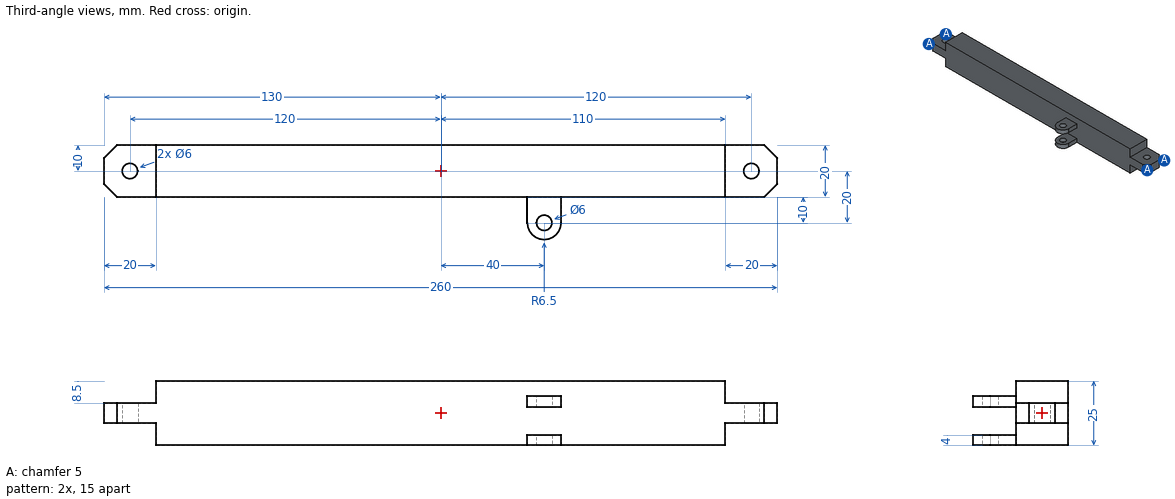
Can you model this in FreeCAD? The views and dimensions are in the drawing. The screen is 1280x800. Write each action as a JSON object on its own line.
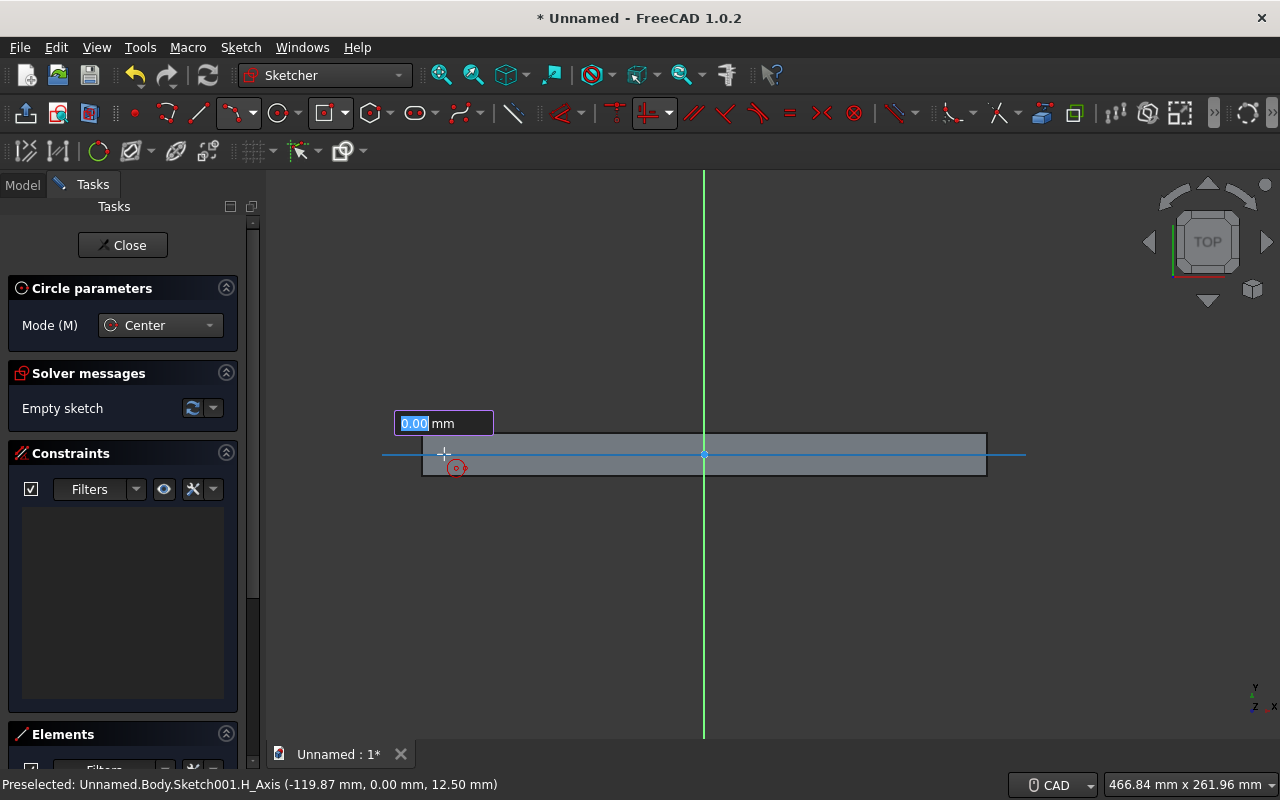
{"action": "scroll", "coordinate": [441, 461], "scroll_direction": "up", "scroll_amount": 5}
{"action": "mouse_move", "coordinate": [442, 459]}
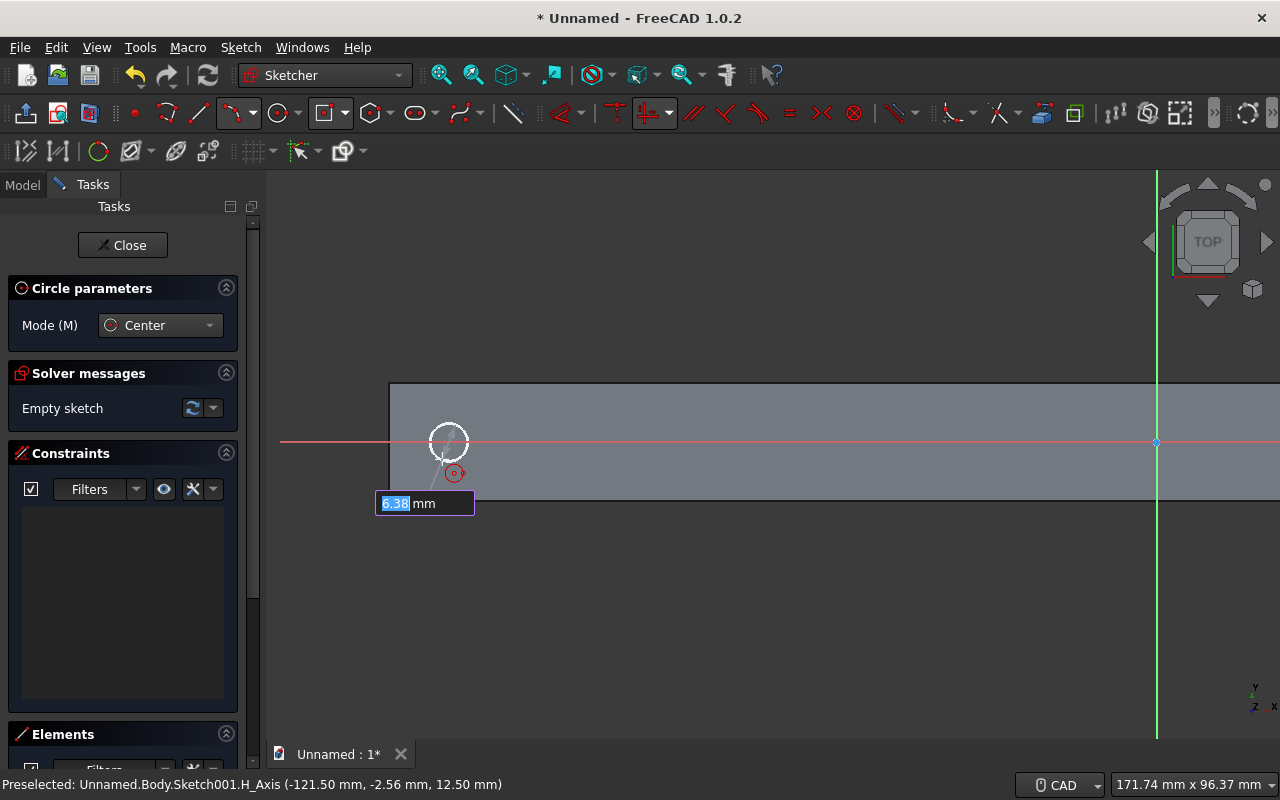
{"action": "type", "text": "6"}
{"action": "key", "text": "Return"}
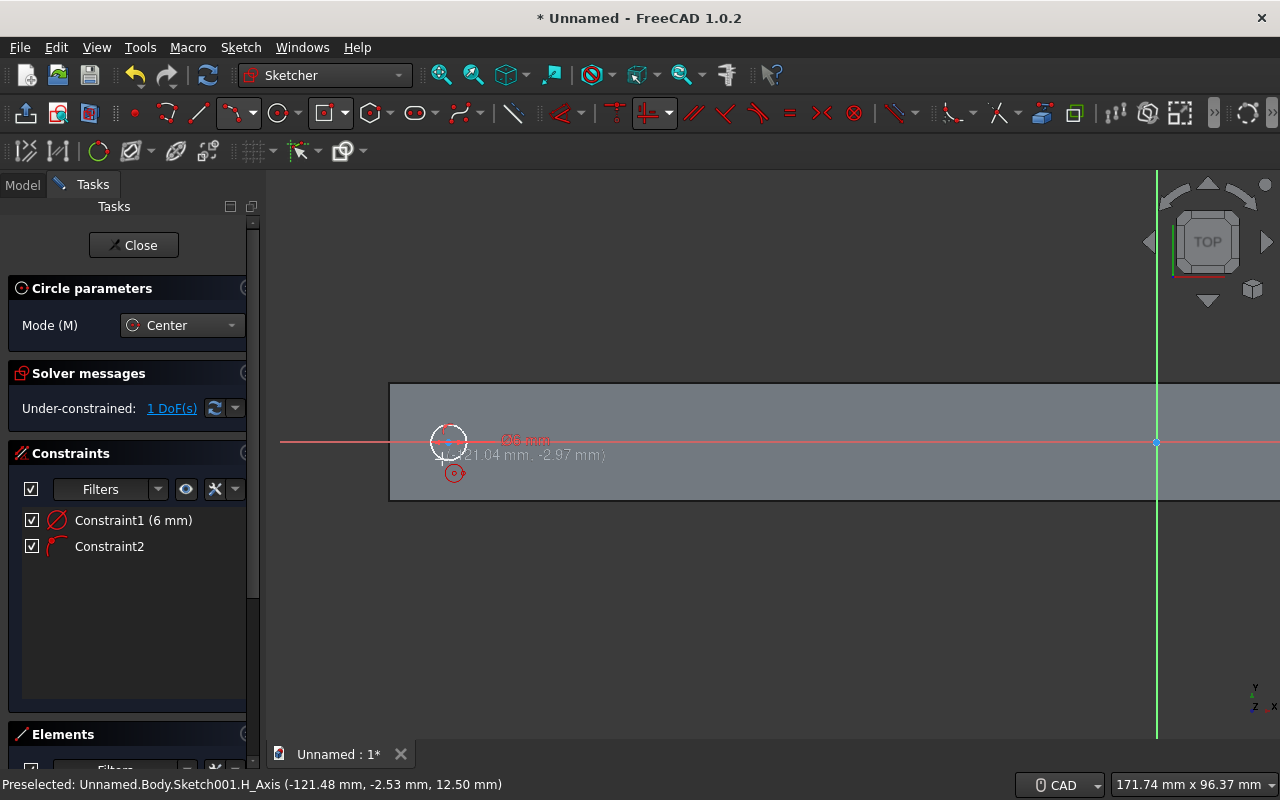
{"action": "scroll", "coordinate": [441, 462], "scroll_direction": "down", "scroll_amount": 5}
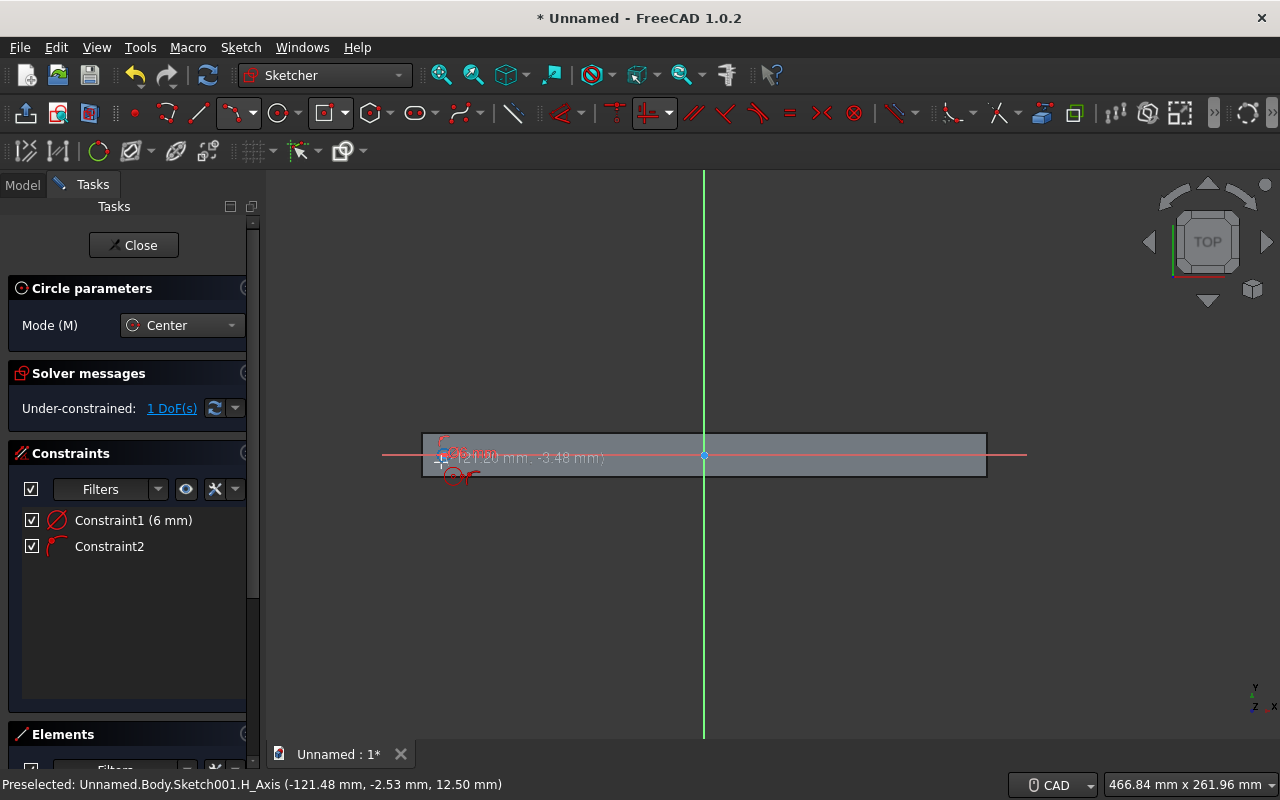
{"action": "scroll", "coordinate": [965, 455], "scroll_direction": "up", "scroll_amount": 7}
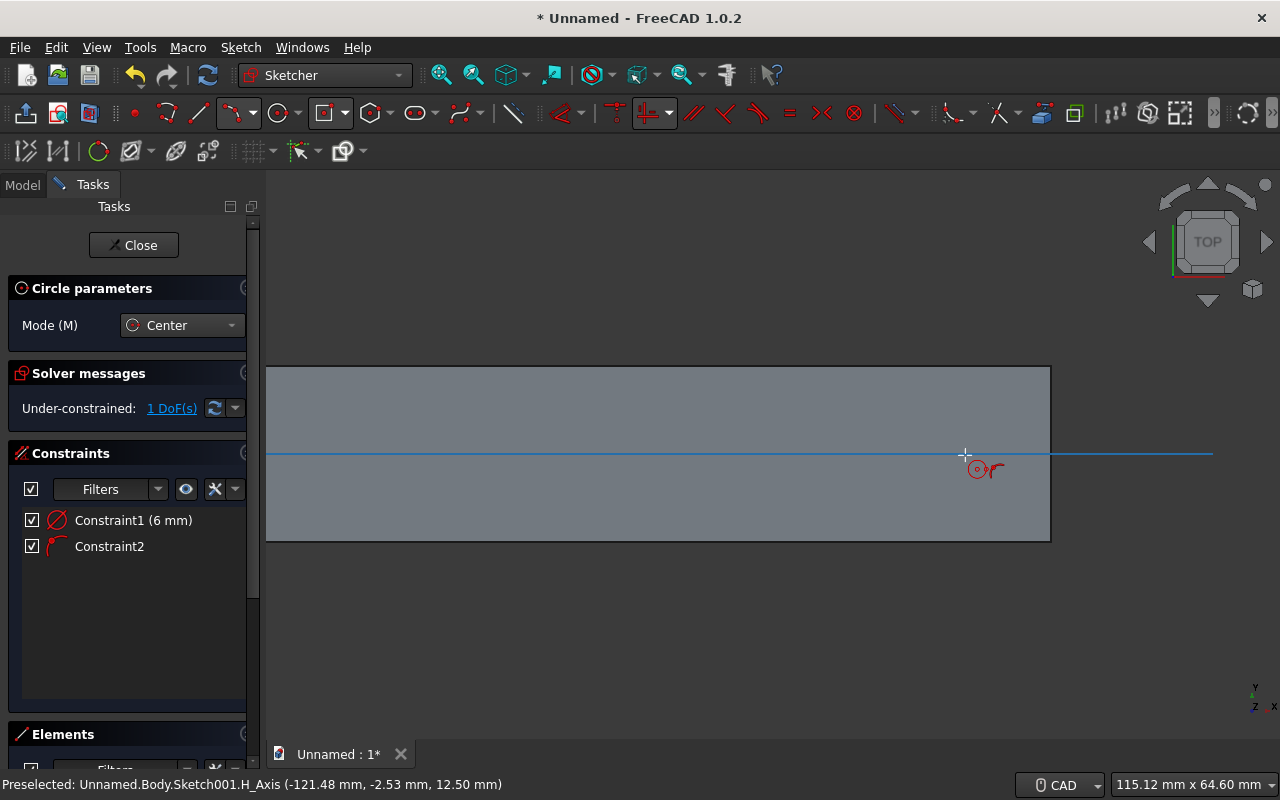
{"action": "scroll", "coordinate": [966, 455], "scroll_direction": "down", "scroll_amount": 7}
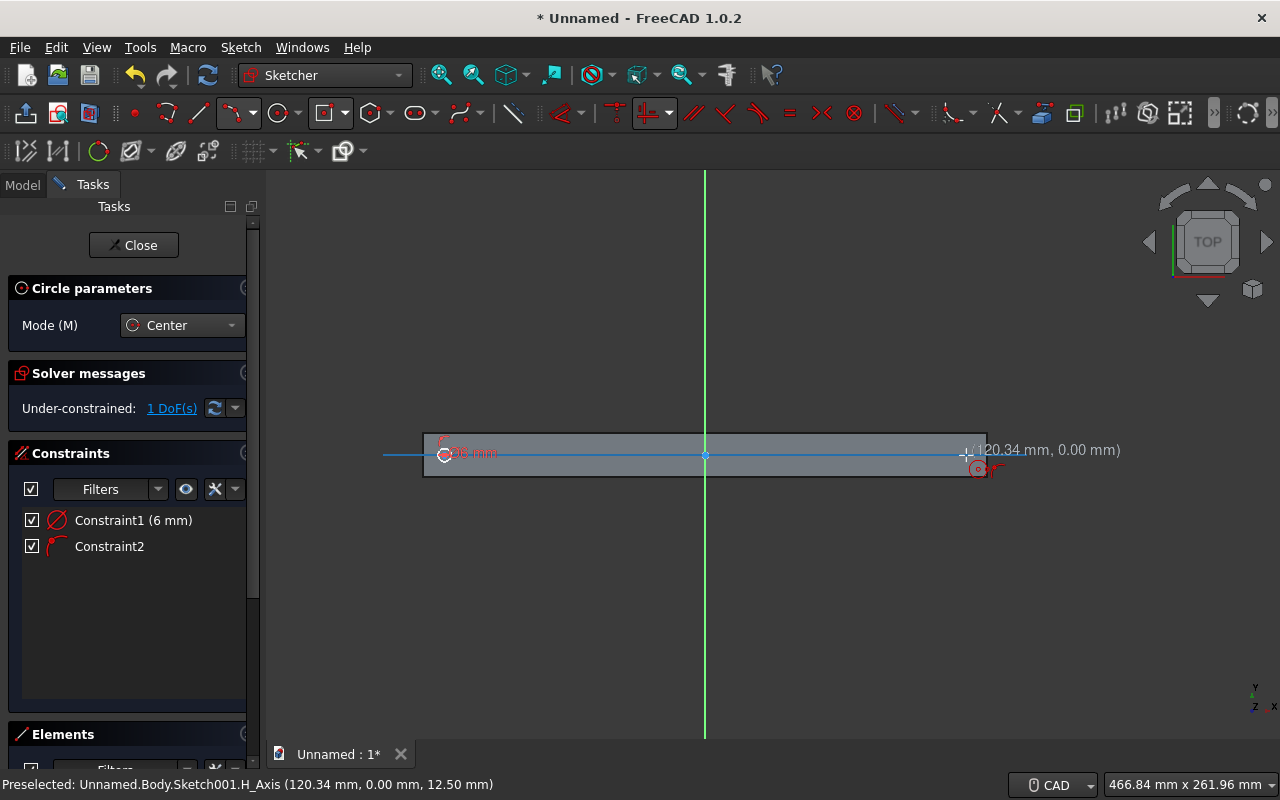
{"action": "left_click", "coordinate": [966, 455]}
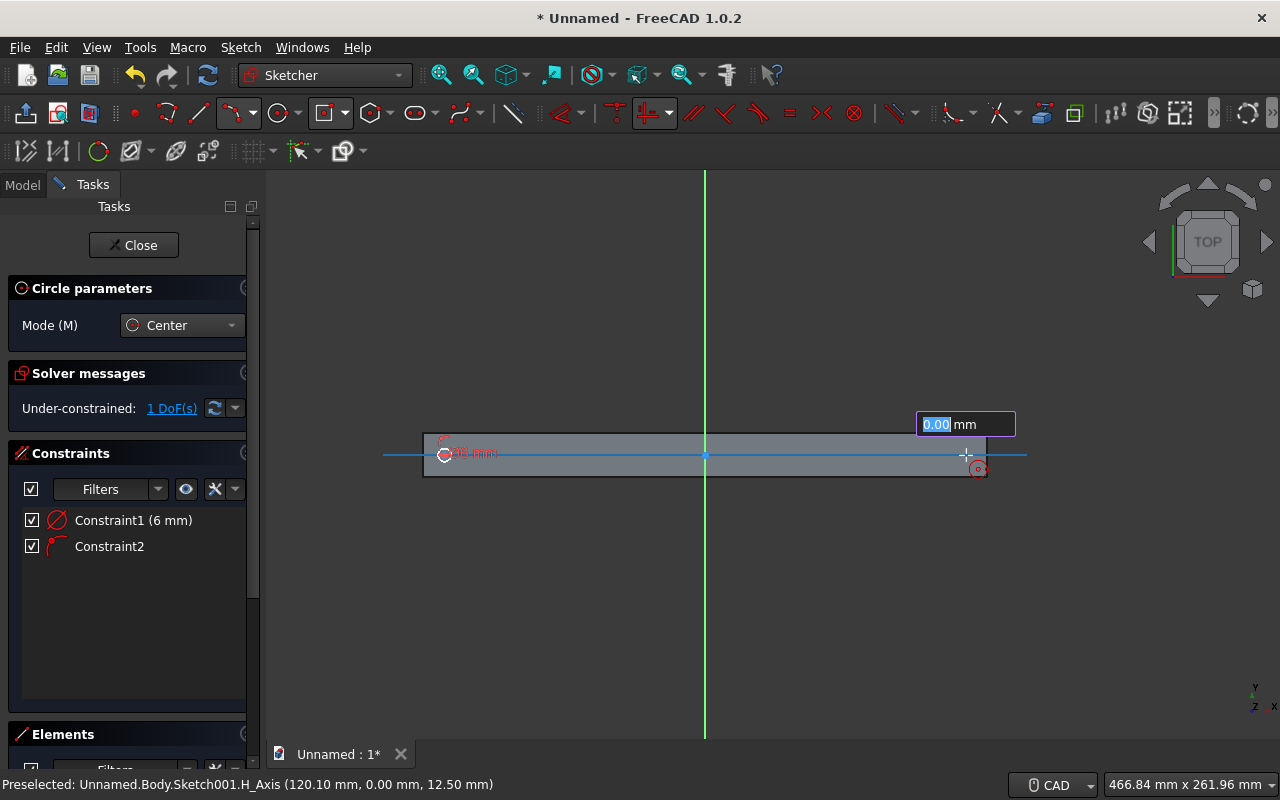
{"action": "scroll", "coordinate": [964, 461], "scroll_direction": "up", "scroll_amount": 5}
{"action": "mouse_move", "coordinate": [962, 461]}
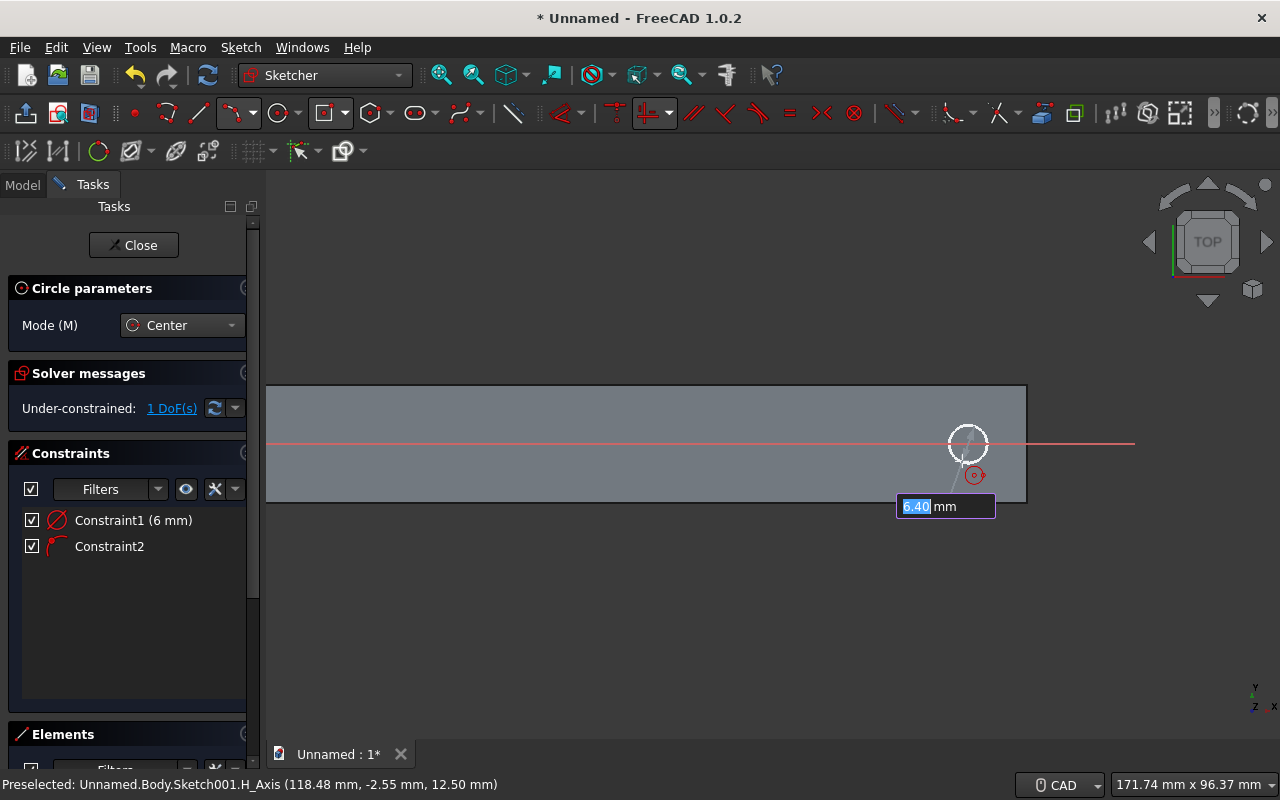
{"action": "type", "text": "6"}
{"action": "key", "text": "Return"}
{"action": "key", "text": "Escape"}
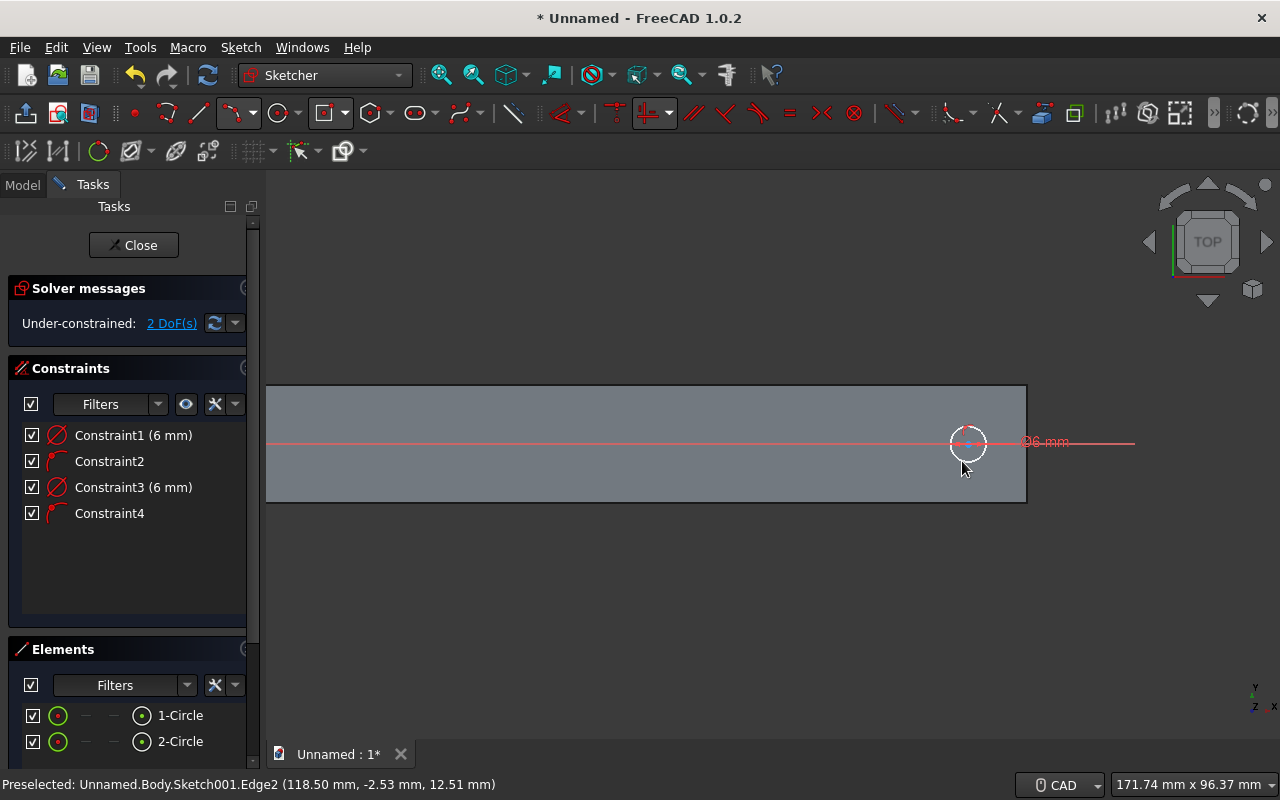
{"action": "left_click", "coordinate": [560, 114]}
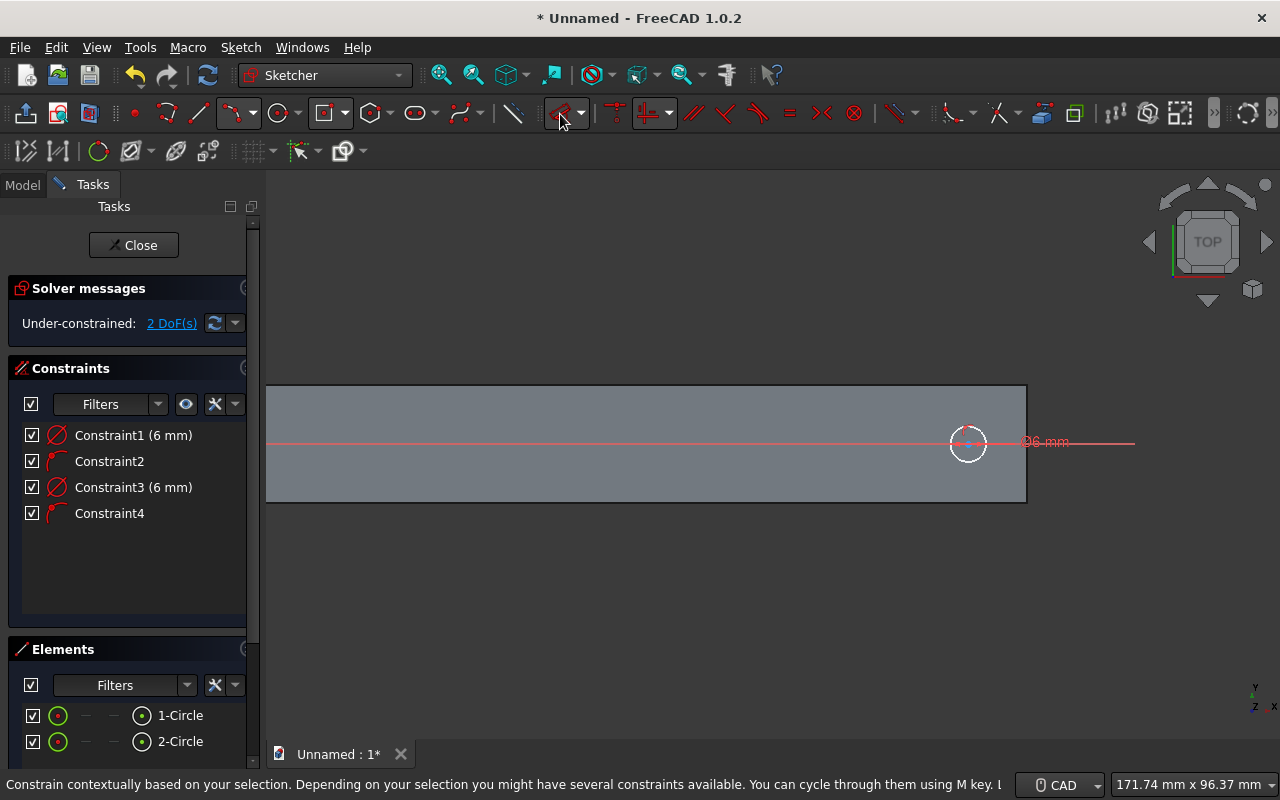
{"action": "scroll", "coordinate": [964, 461], "scroll_direction": "down", "scroll_amount": 5}